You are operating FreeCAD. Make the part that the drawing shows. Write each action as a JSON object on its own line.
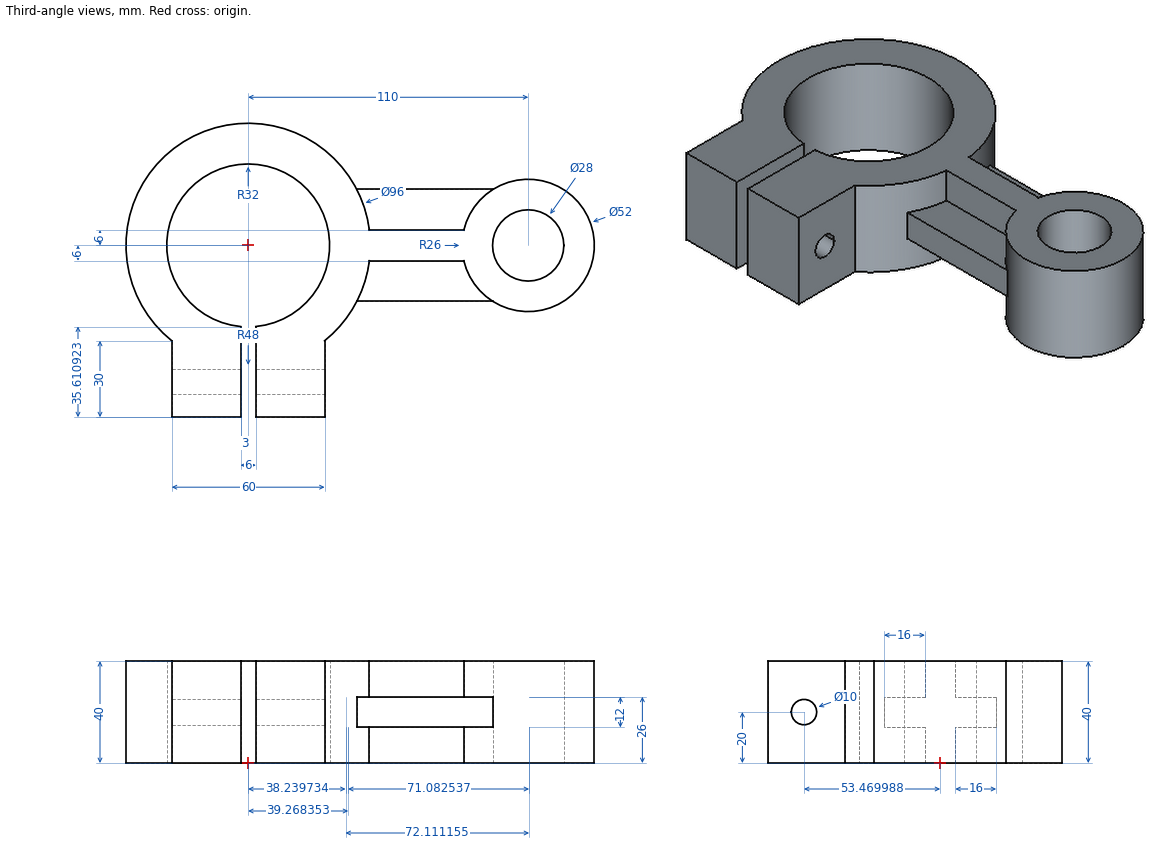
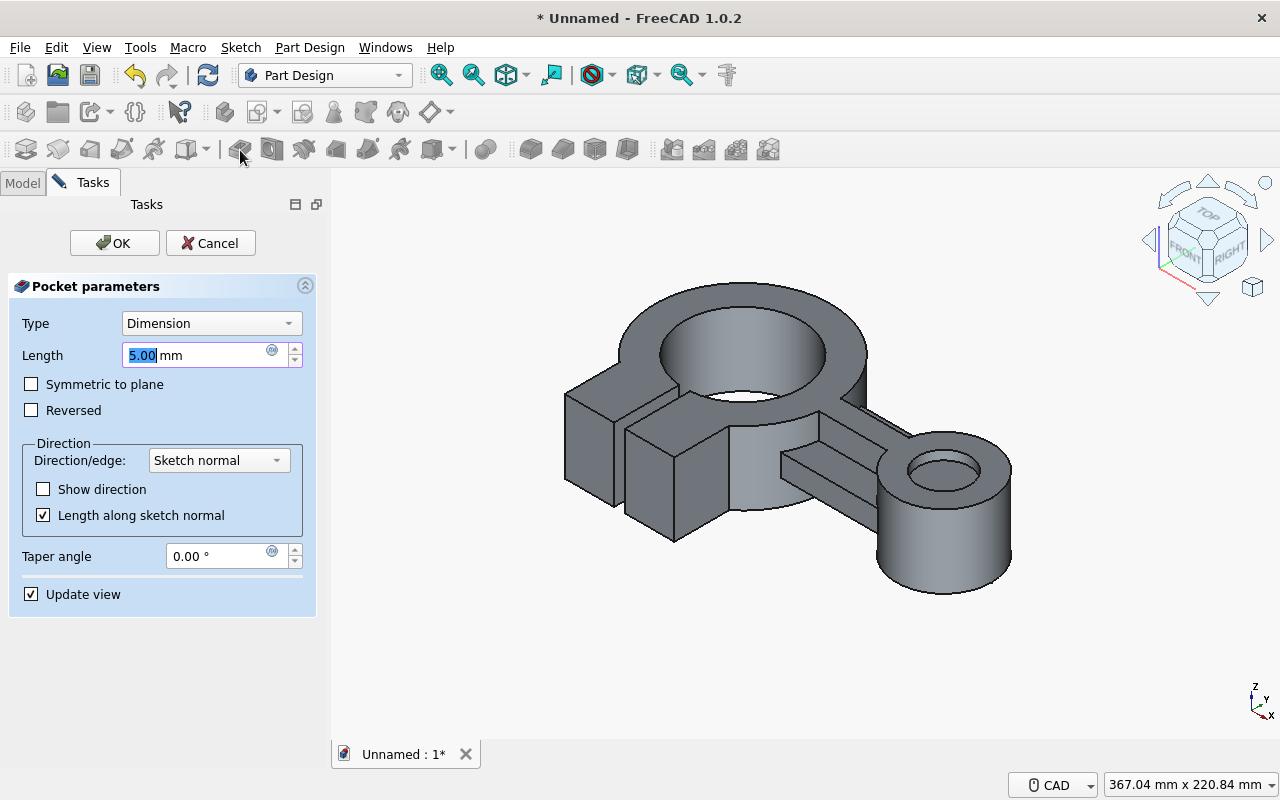
{"action": "type", "text": "40"}
{"action": "key", "text": "Tab"}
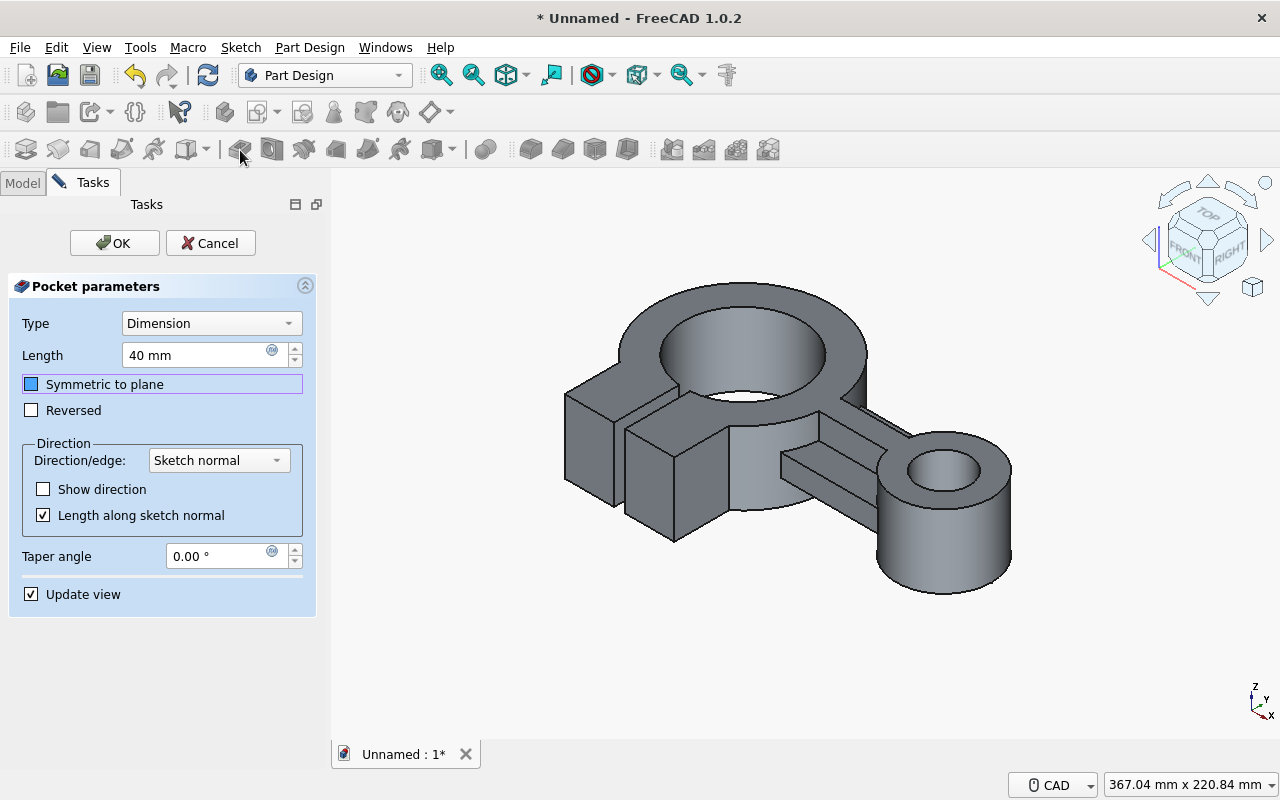
{"action": "left_click", "coordinate": [115, 243]}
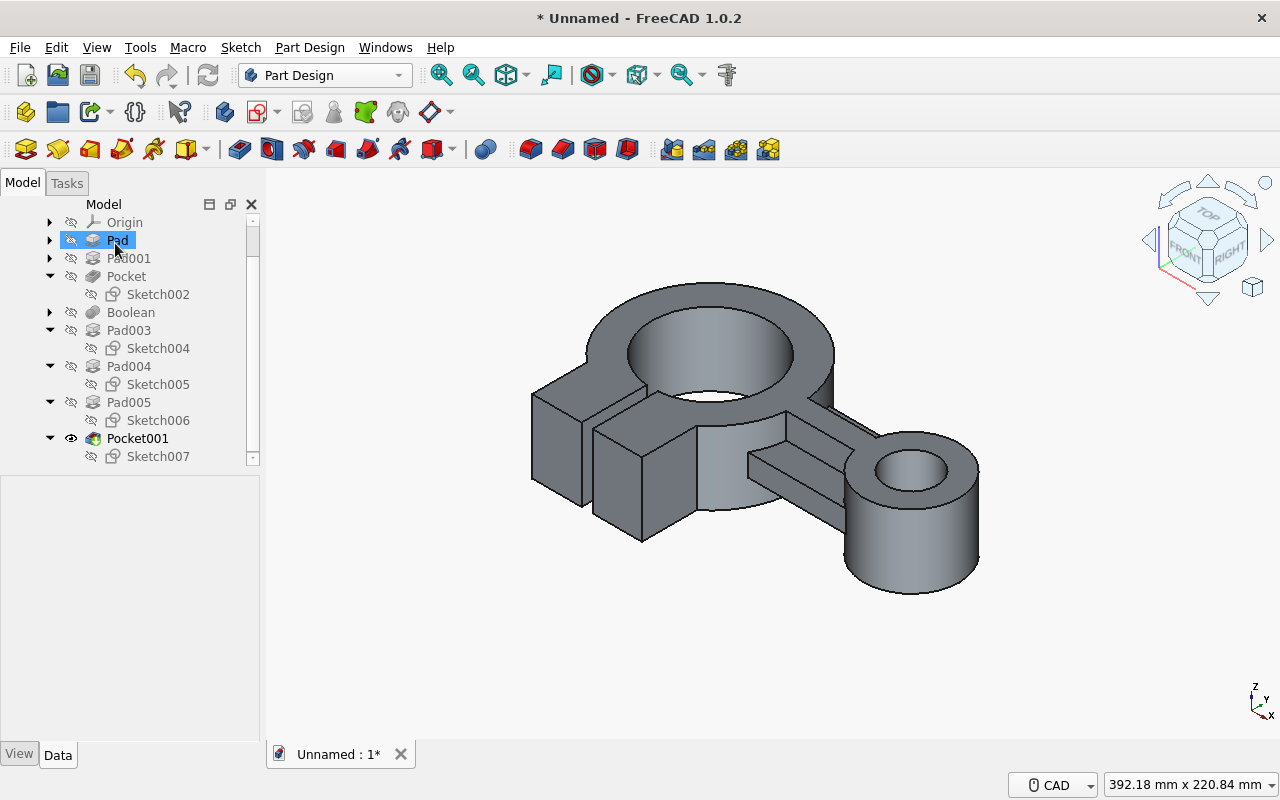
{"action": "left_click", "coordinate": [669, 483]}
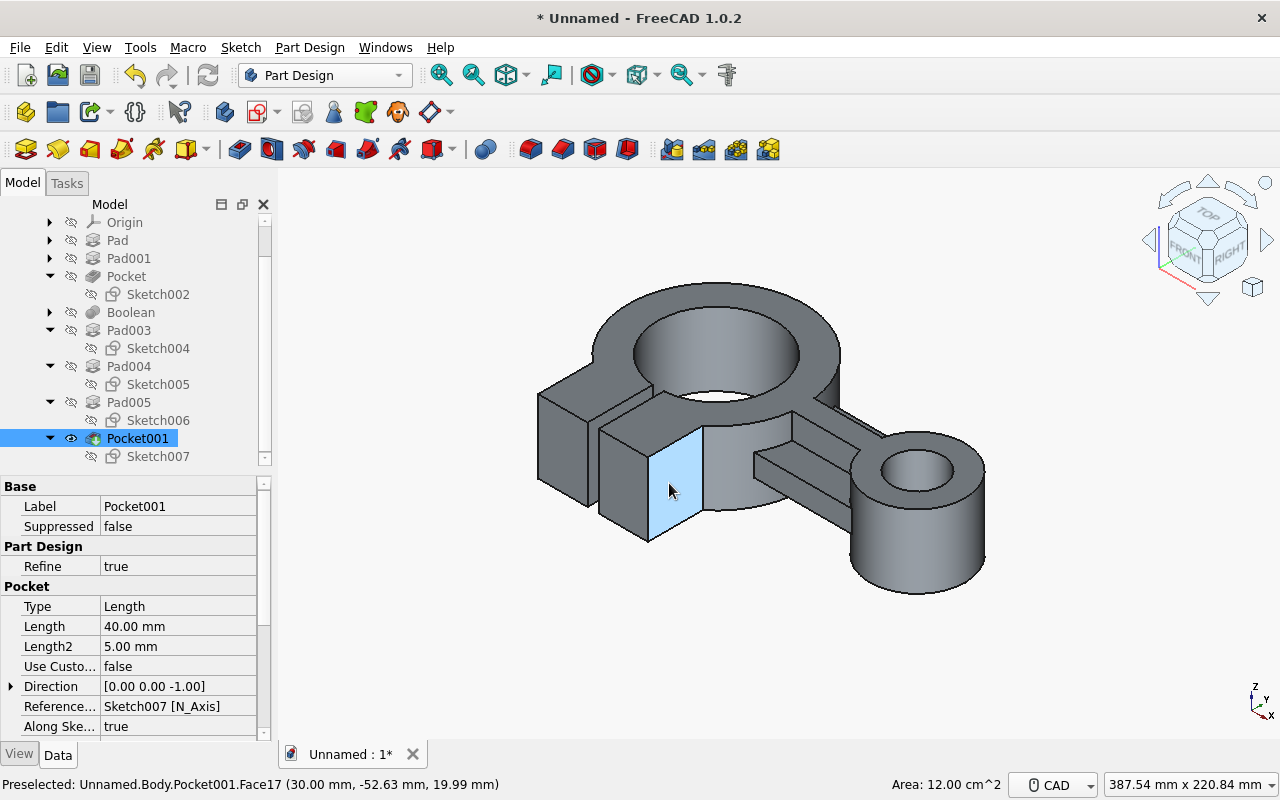
{"action": "left_click", "coordinate": [258, 112]}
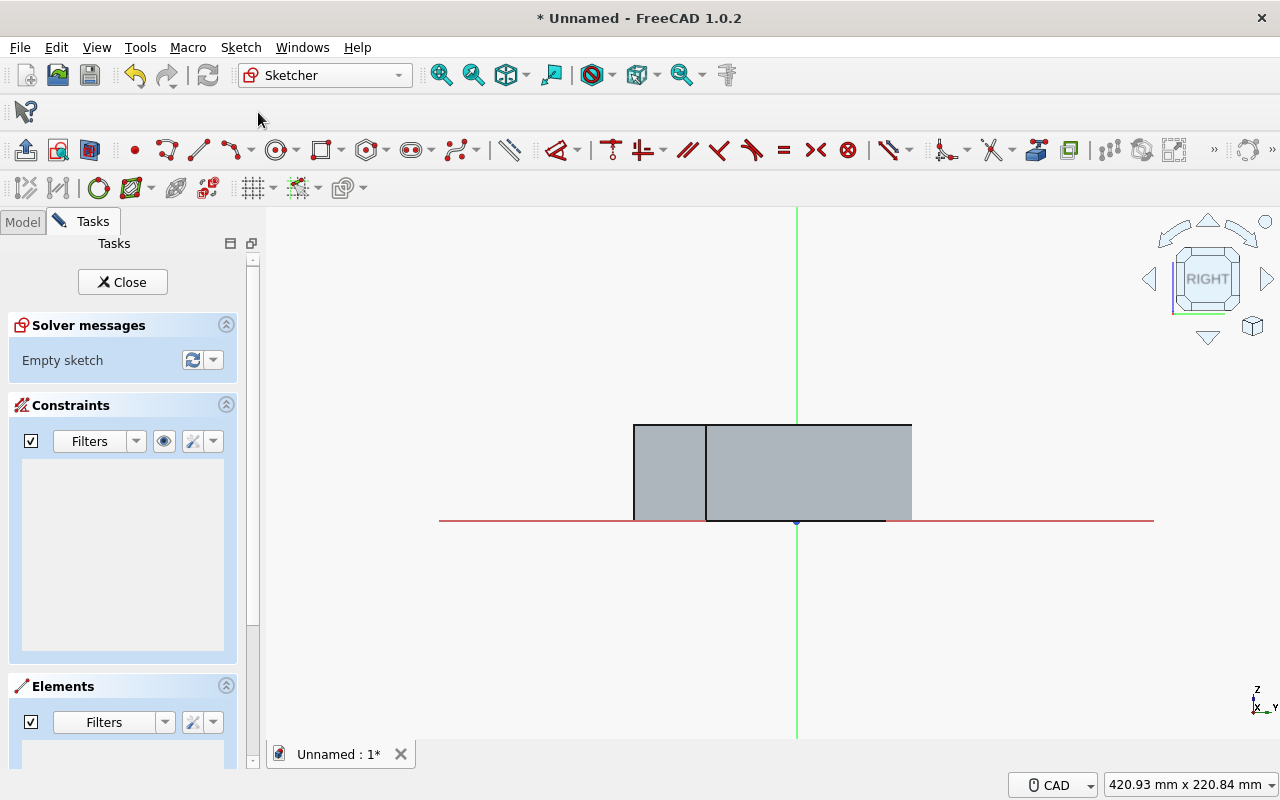
{"action": "scroll", "coordinate": [665, 473], "scroll_direction": "up", "scroll_amount": 13}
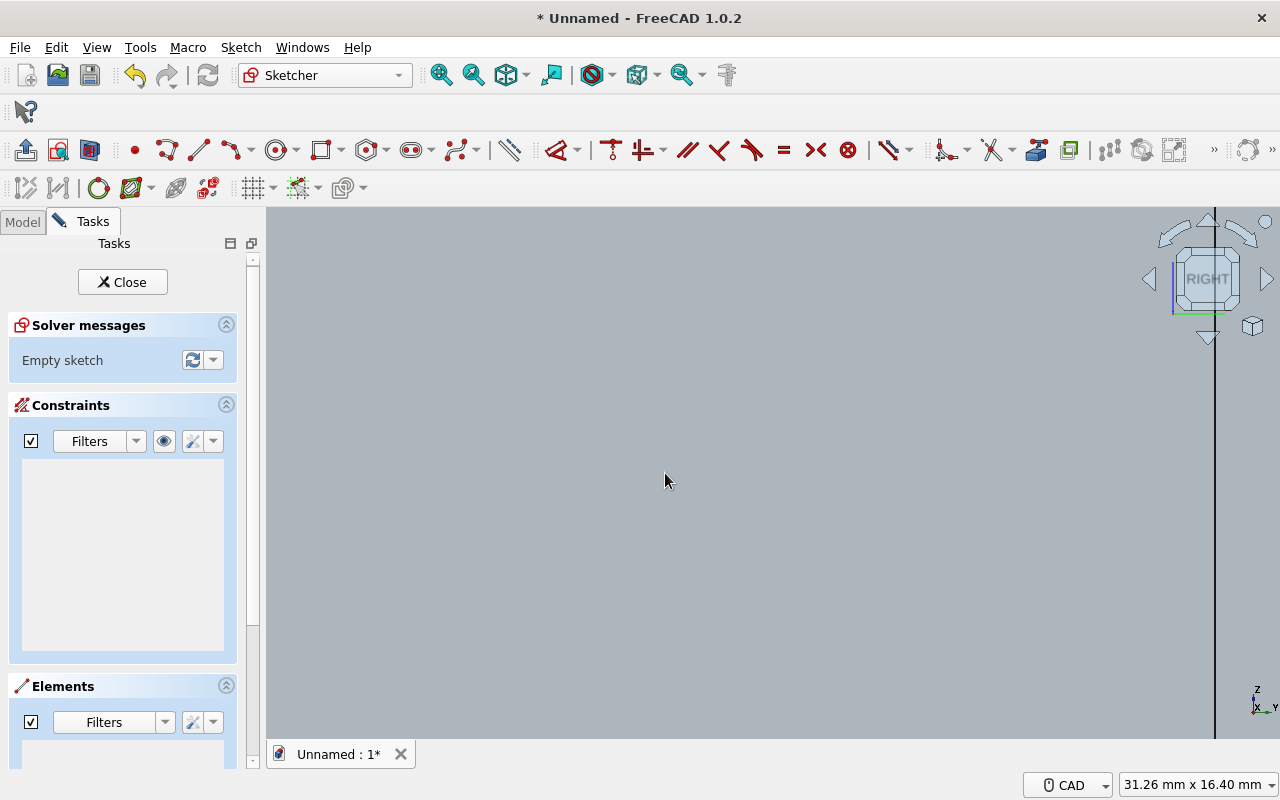
{"action": "left_click", "coordinate": [276, 150]}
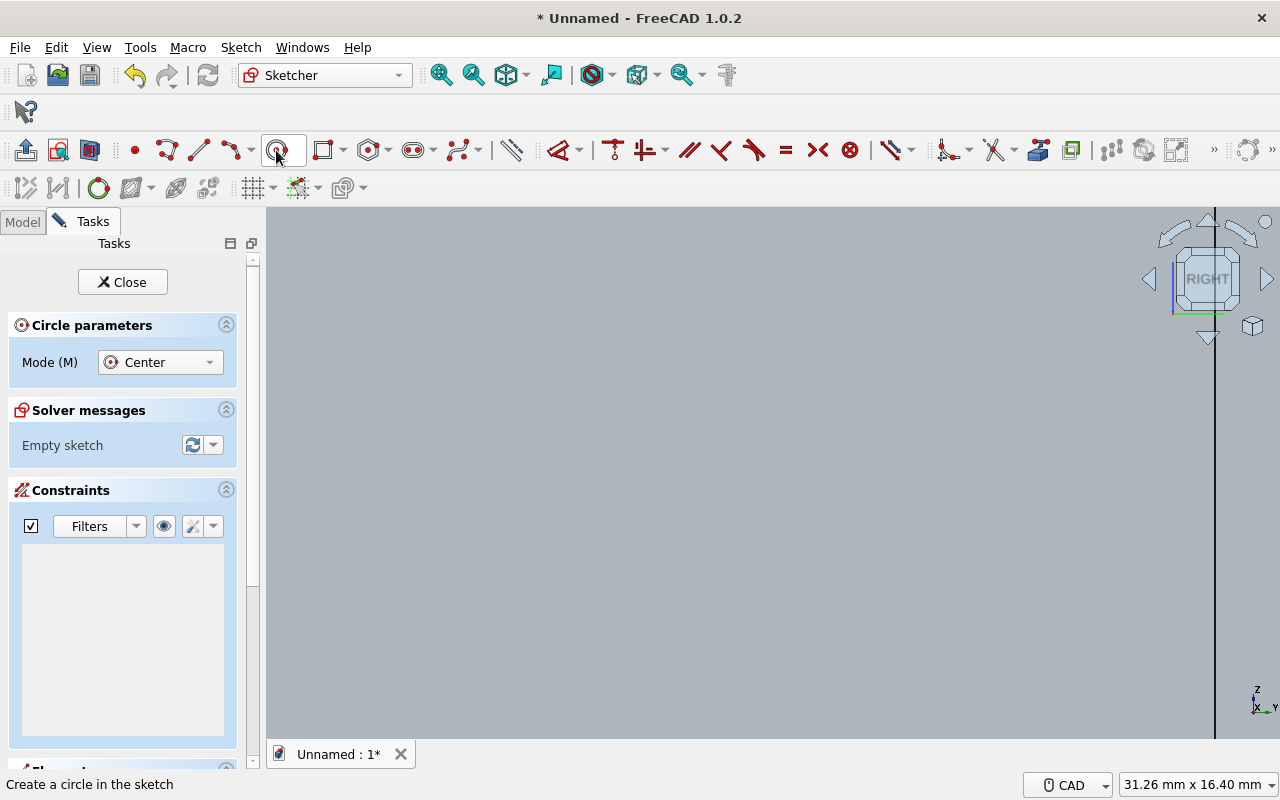
{"action": "left_click", "coordinate": [696, 467]}
{"action": "left_click", "coordinate": [811, 352]}
{"action": "key", "text": "Escape"}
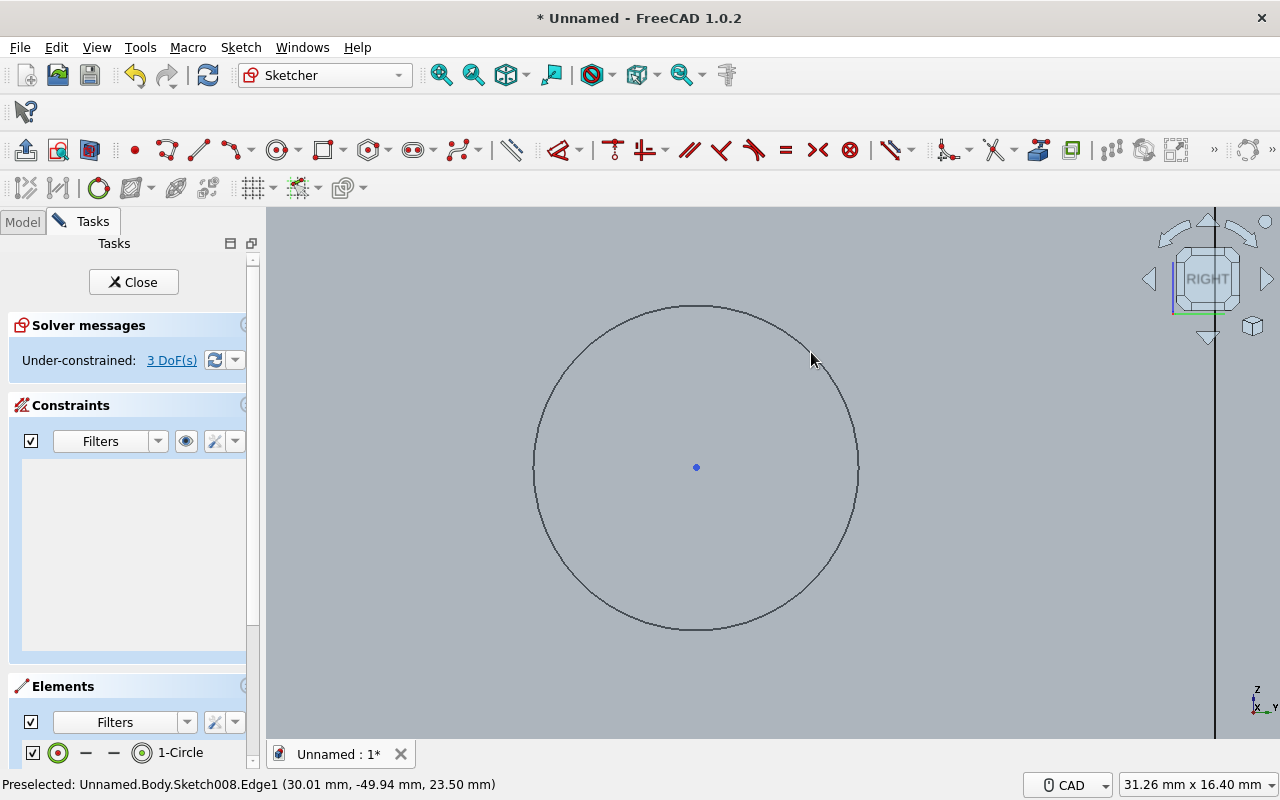
{"action": "left_click", "coordinate": [558, 150]}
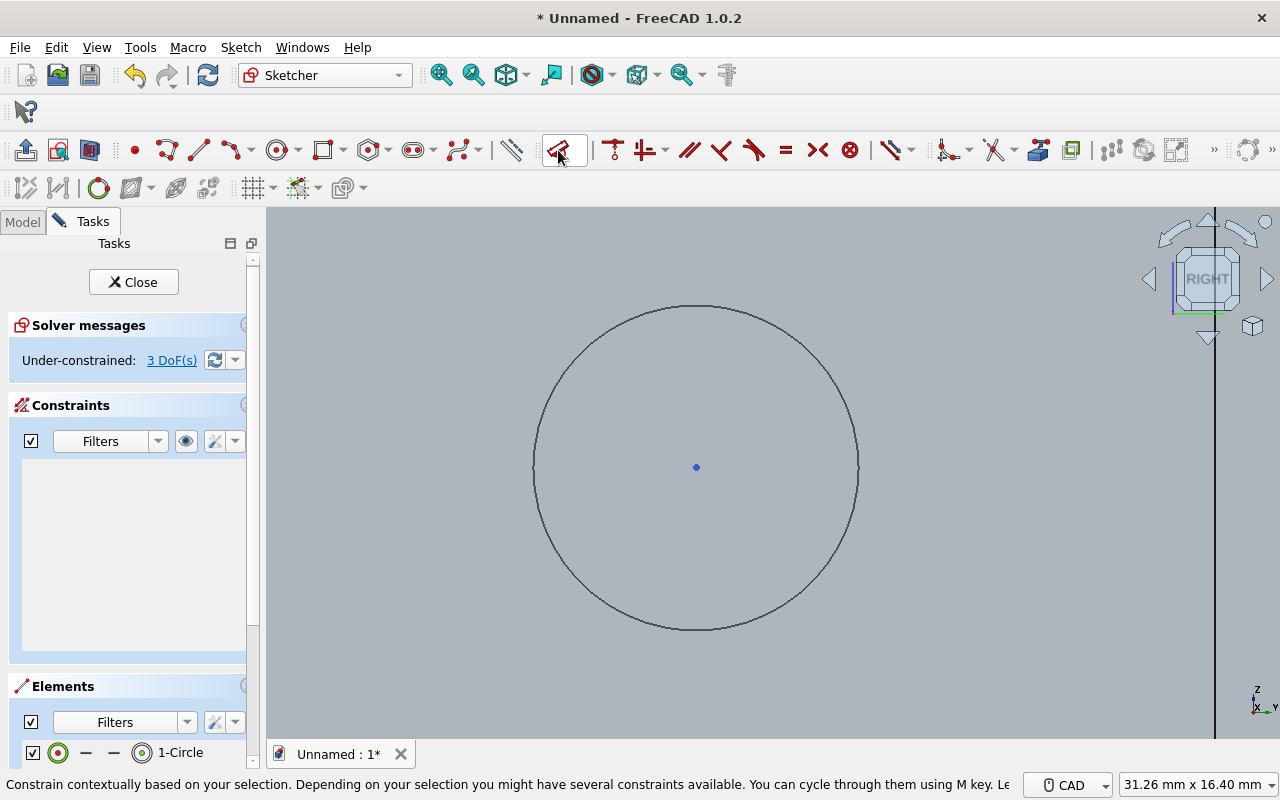
{"action": "left_click", "coordinate": [811, 353]}
{"action": "left_click", "coordinate": [834, 330]}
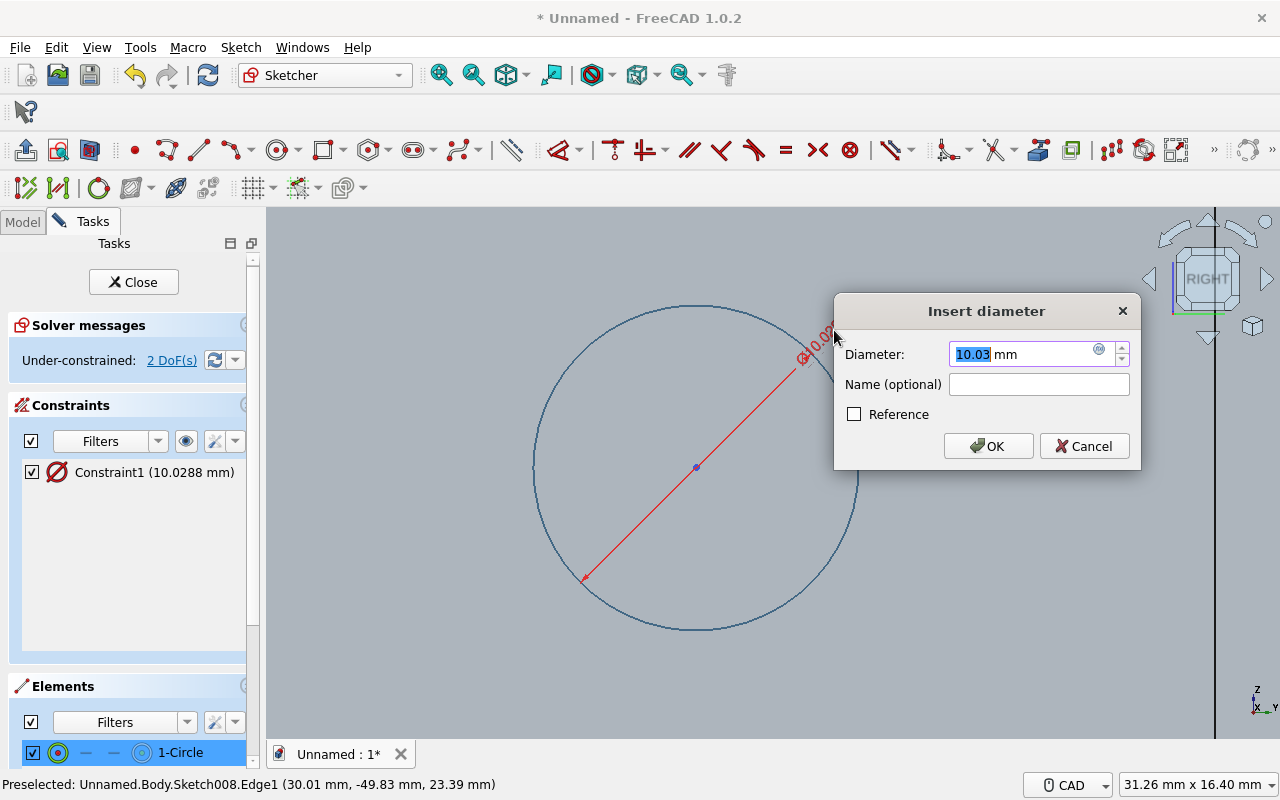
{"action": "type", "text": "10"}
{"action": "key", "text": "Return"}